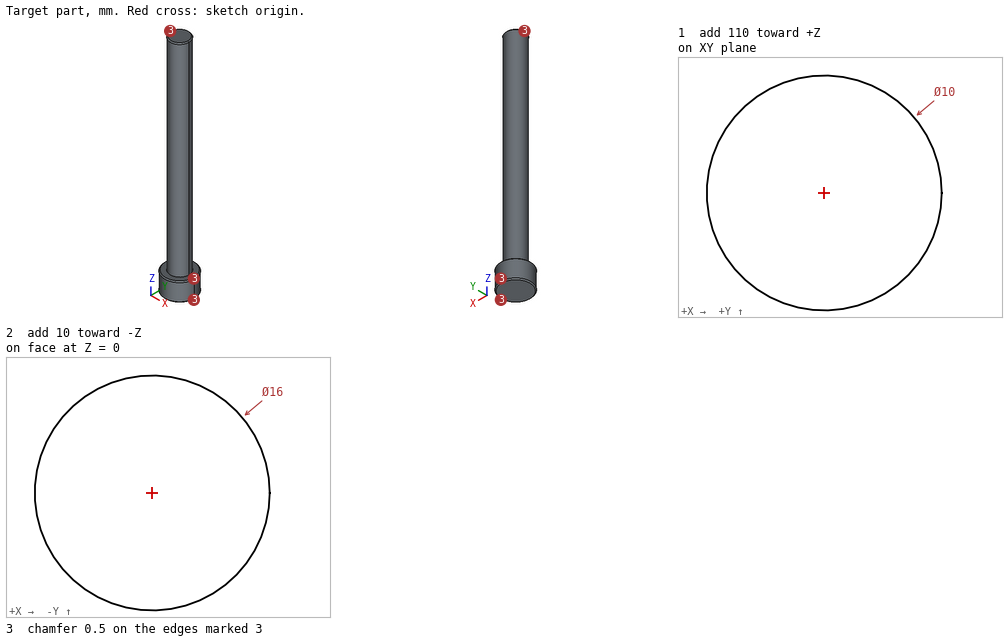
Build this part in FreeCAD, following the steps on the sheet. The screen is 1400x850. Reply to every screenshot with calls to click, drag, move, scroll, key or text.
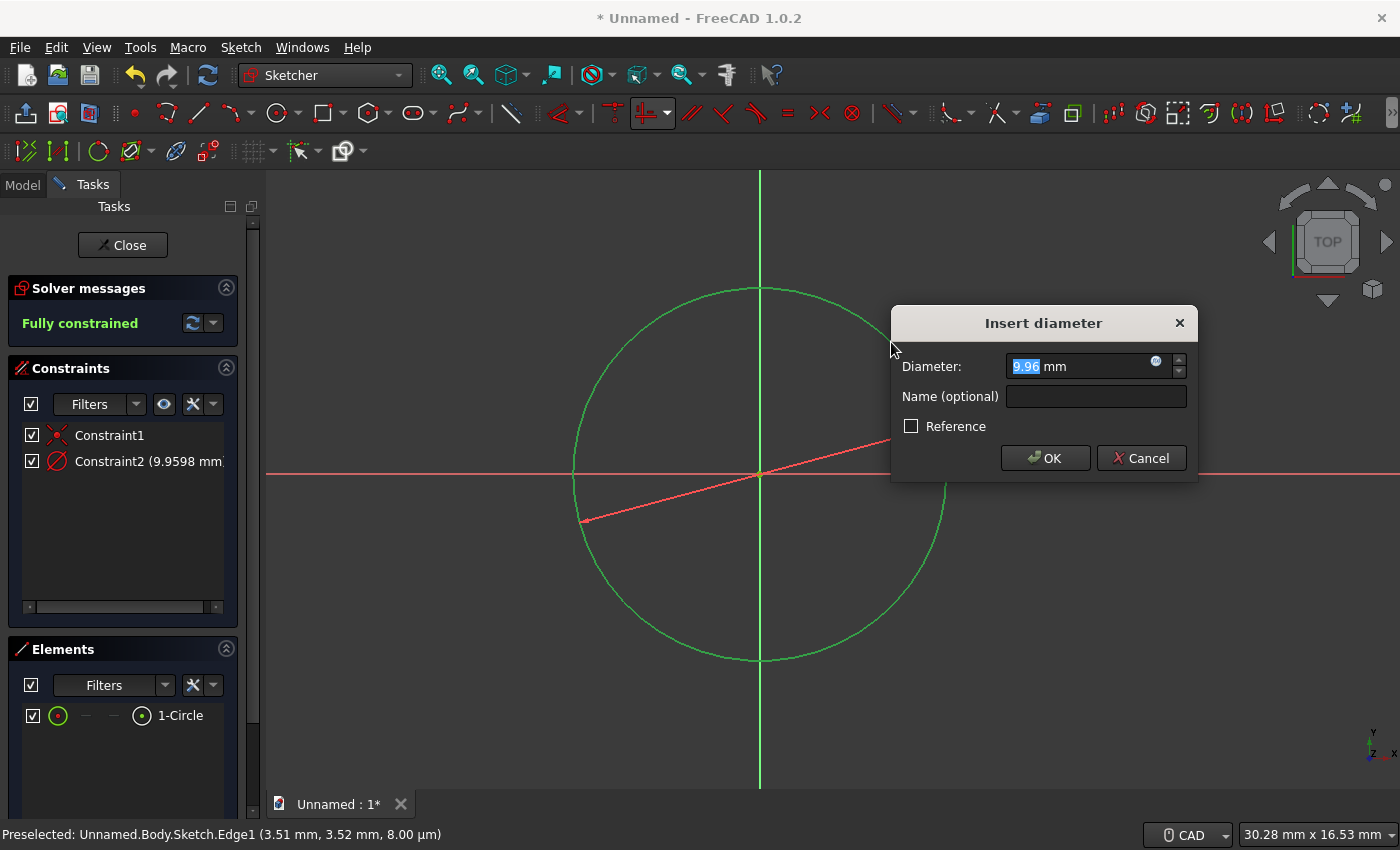
text(10)
key(Return)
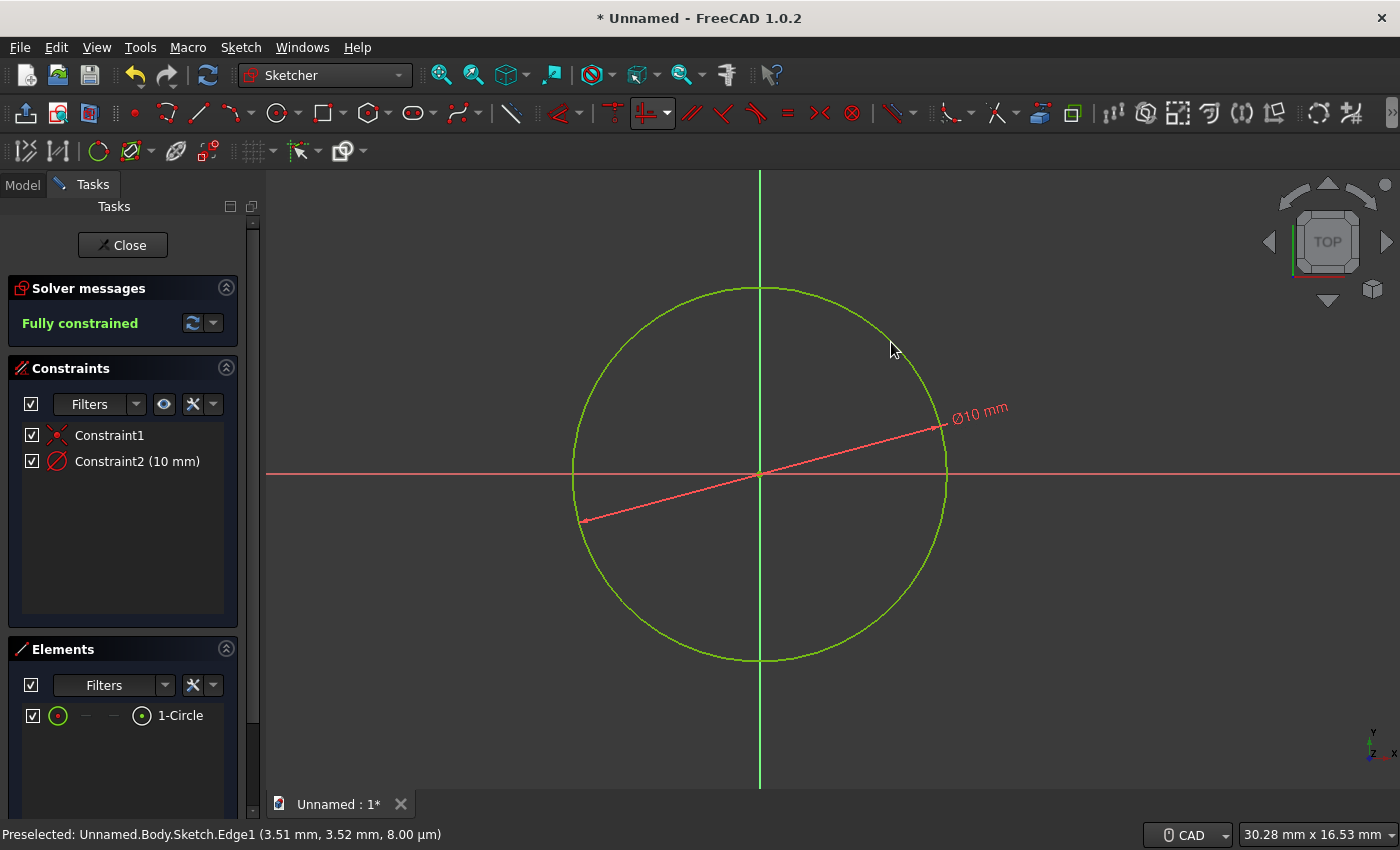
click(123, 245)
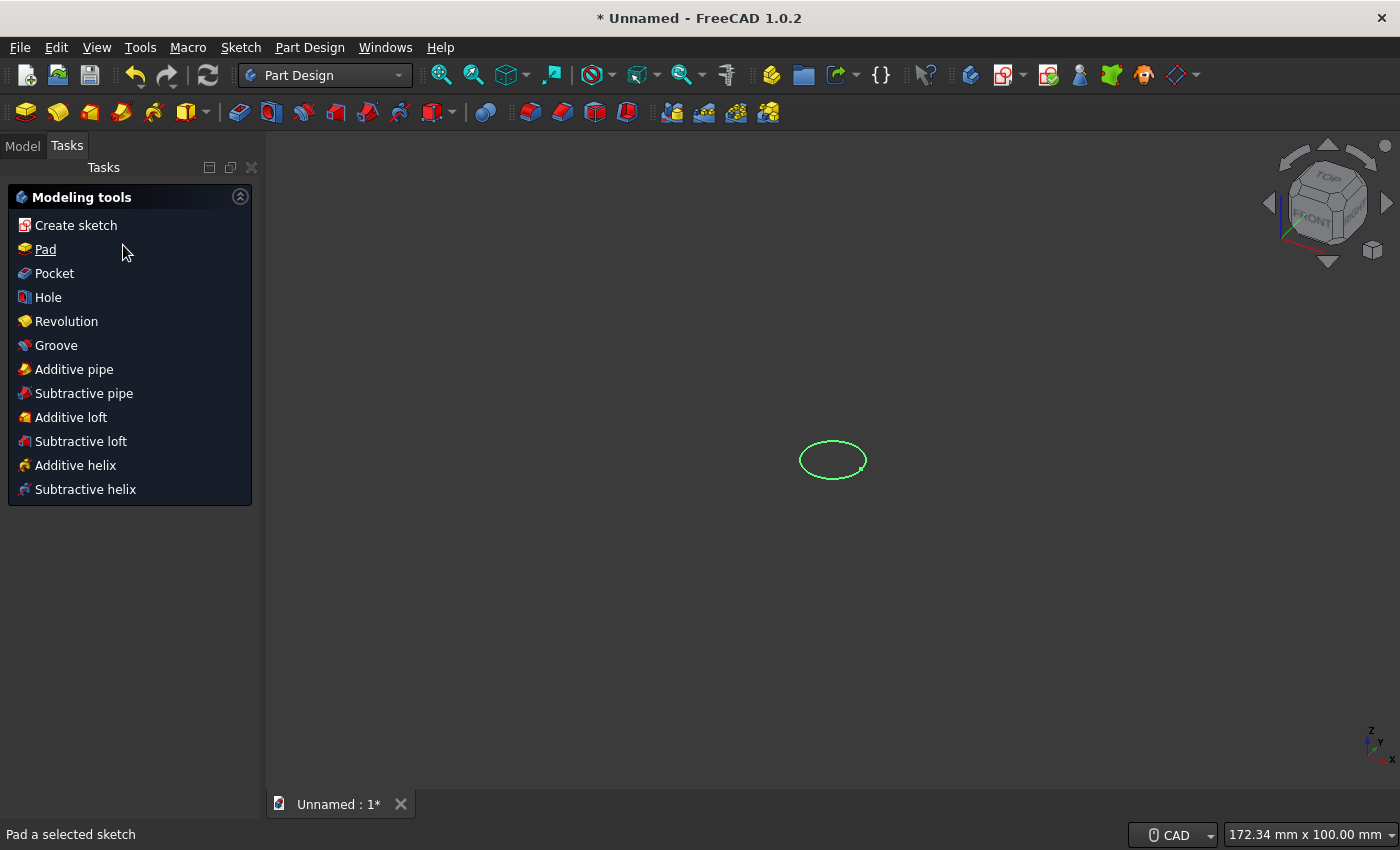
click(26, 112)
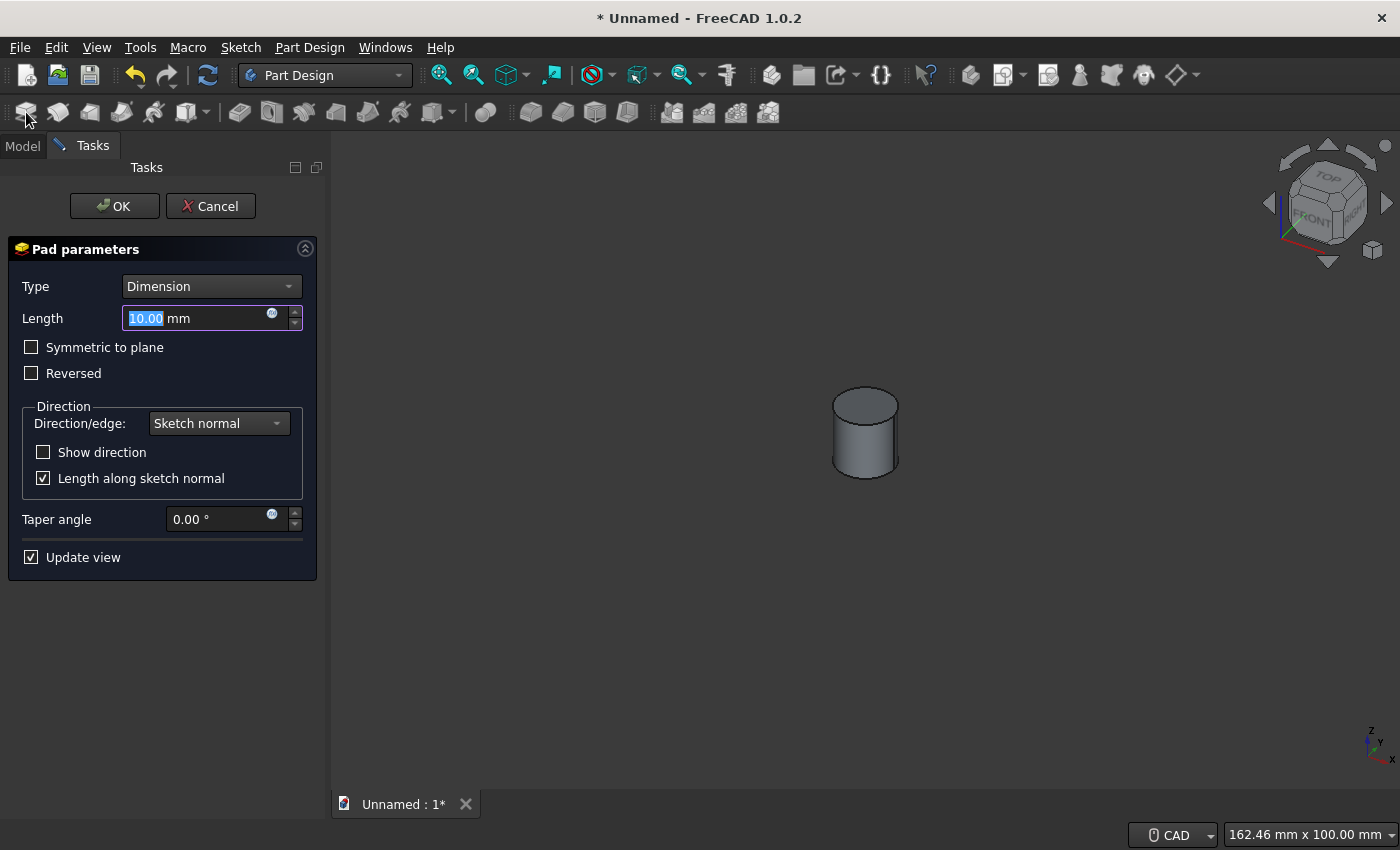
text(110)
key(Tab)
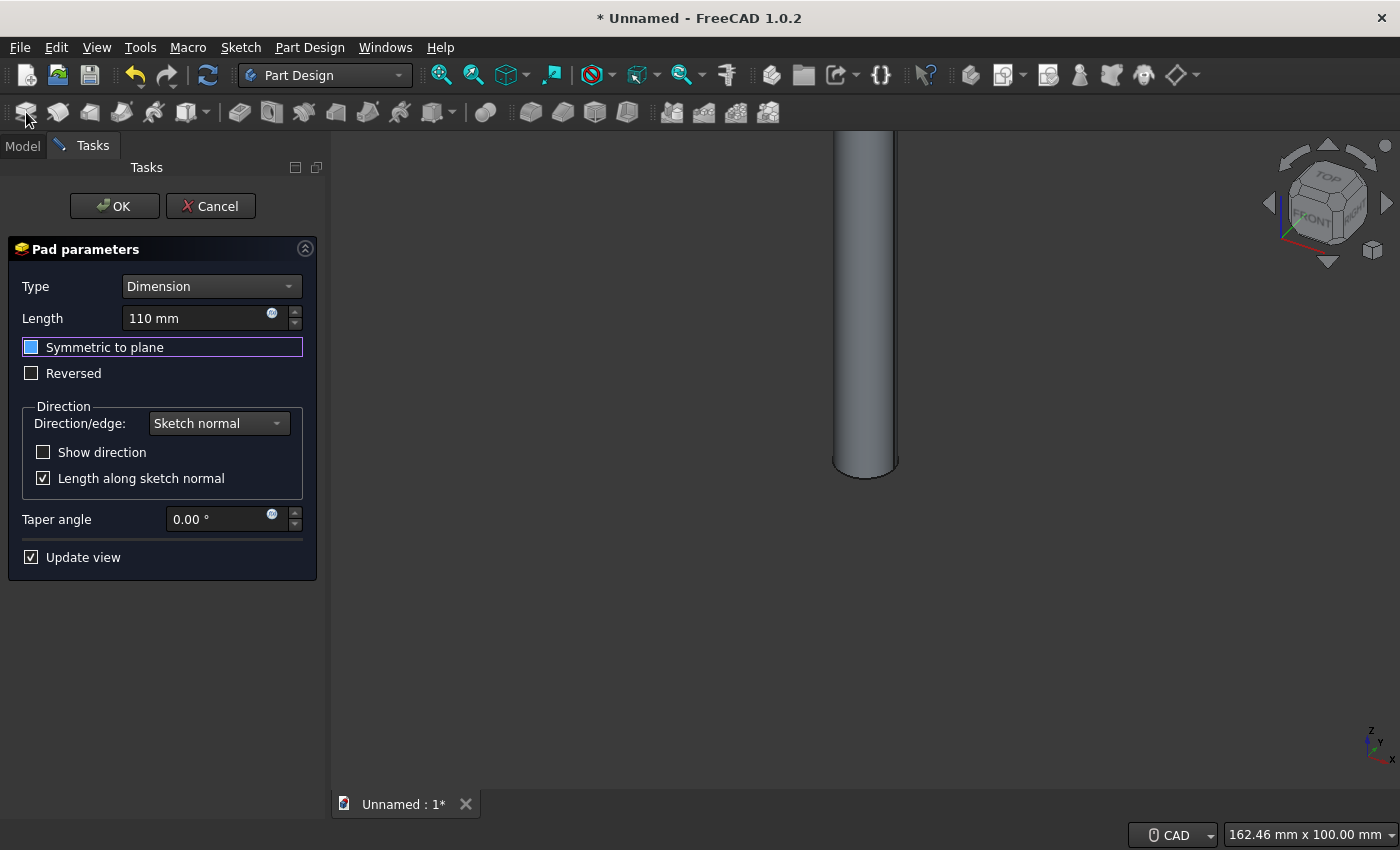
click(115, 206)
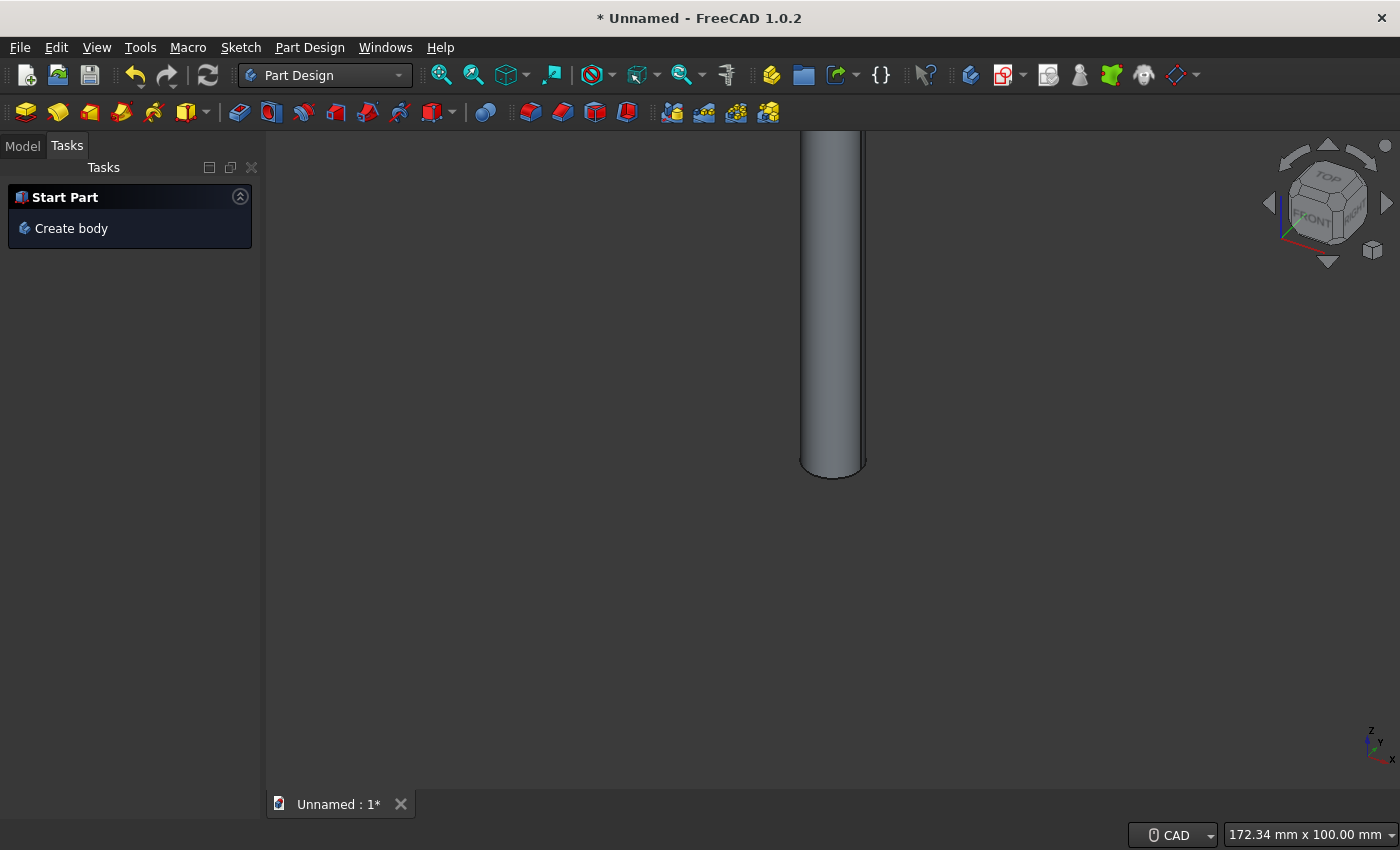
key(v)
key(f)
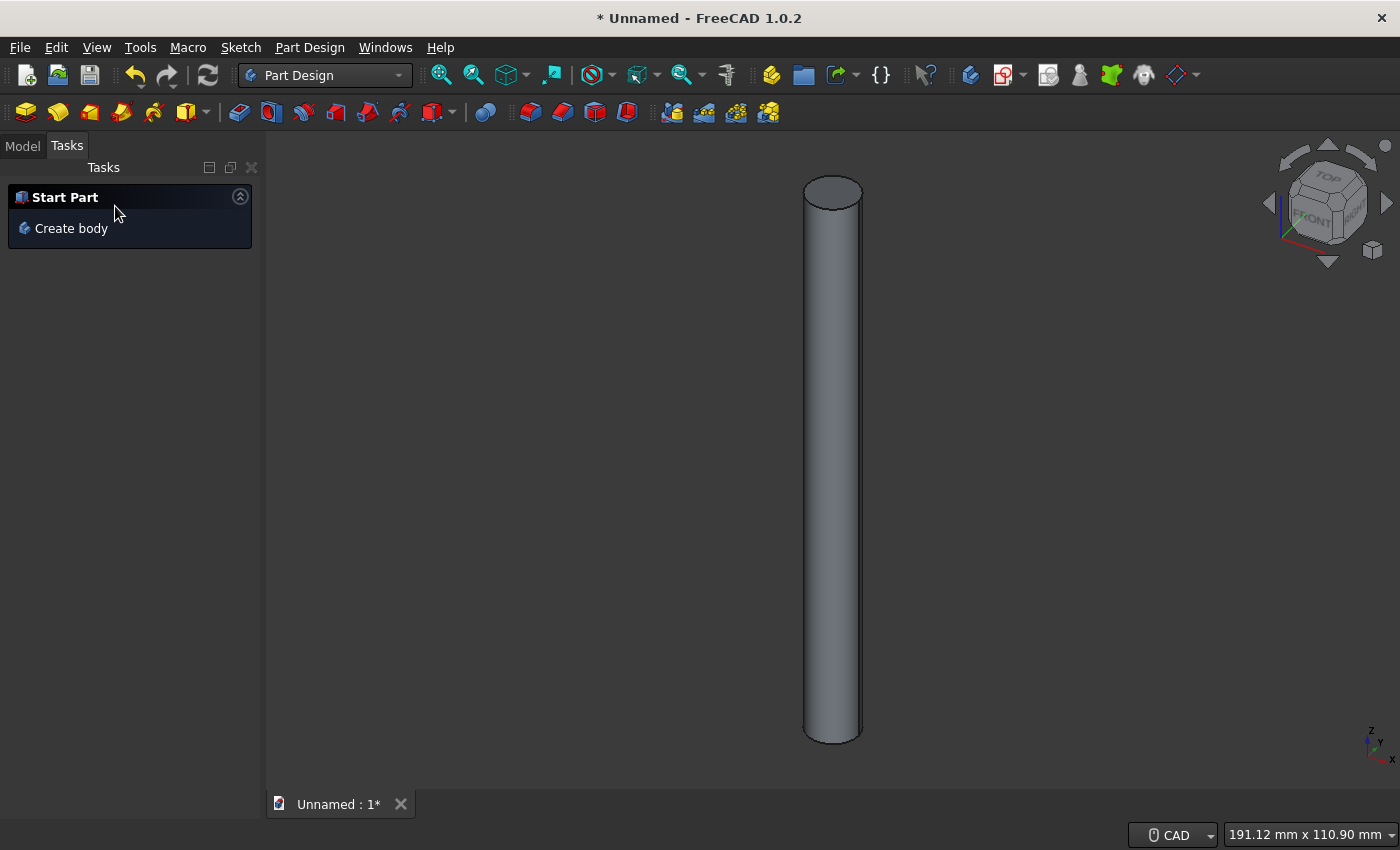
key(5)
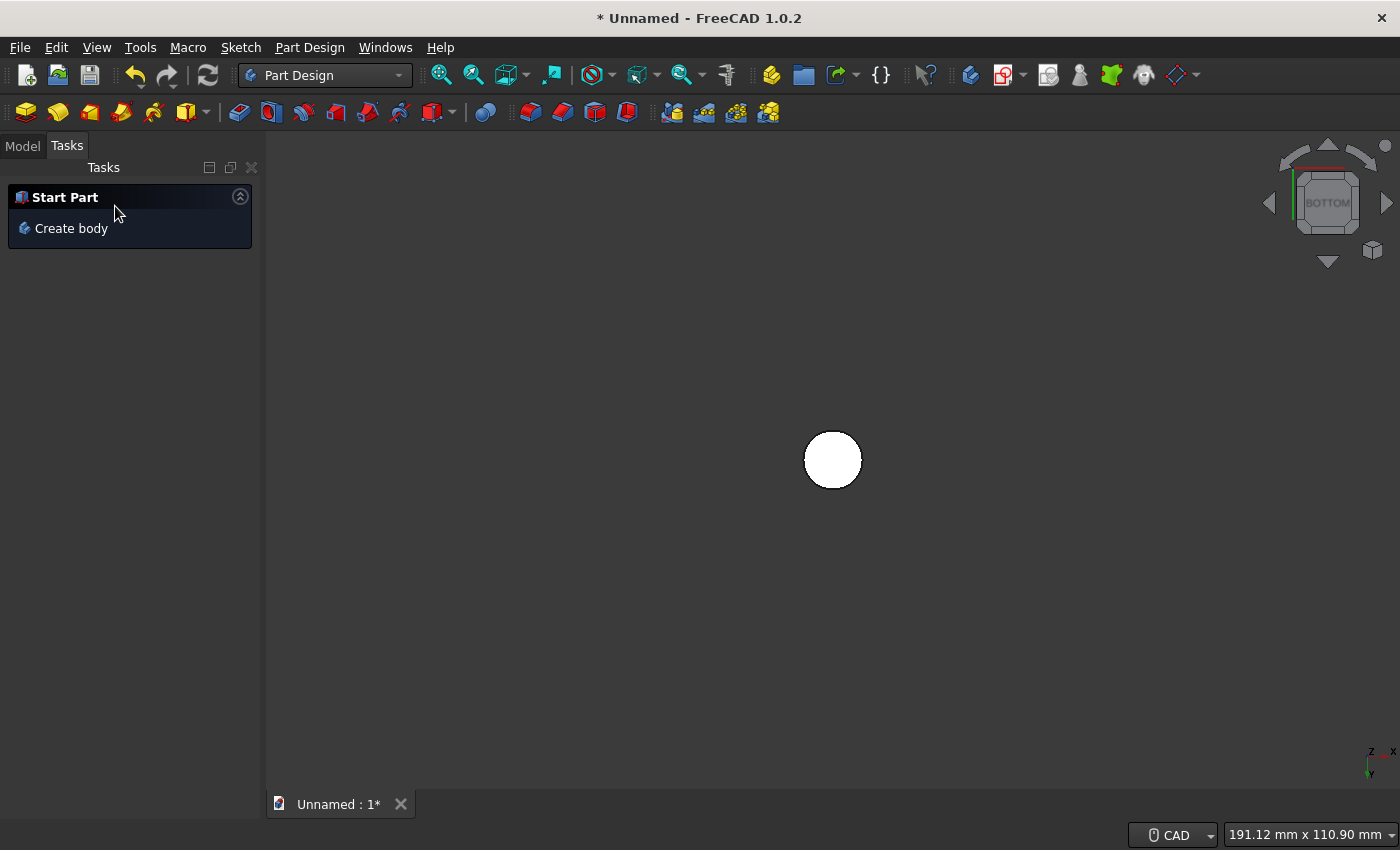
click(442, 76)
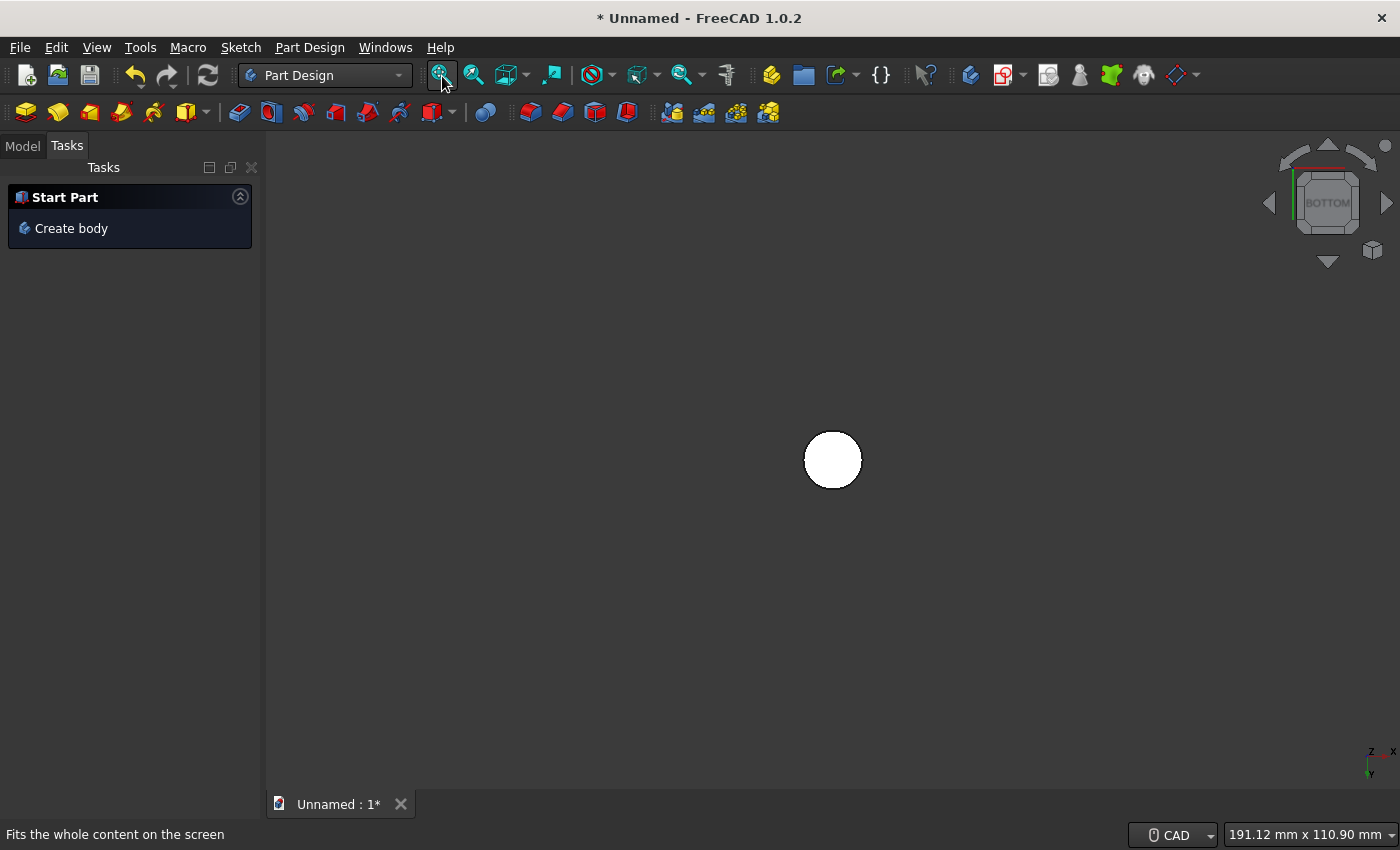
click(833, 459)